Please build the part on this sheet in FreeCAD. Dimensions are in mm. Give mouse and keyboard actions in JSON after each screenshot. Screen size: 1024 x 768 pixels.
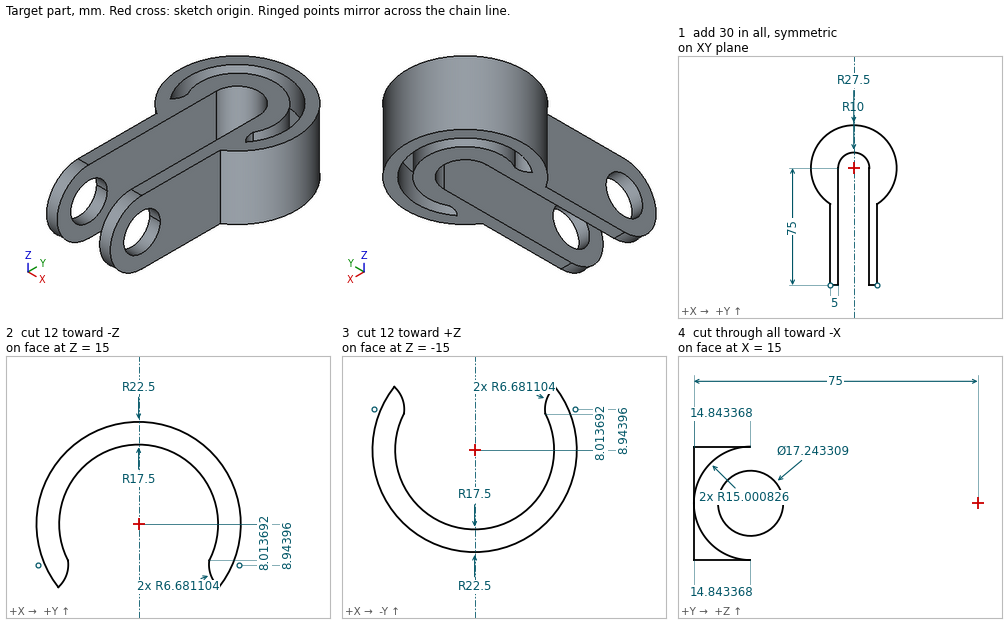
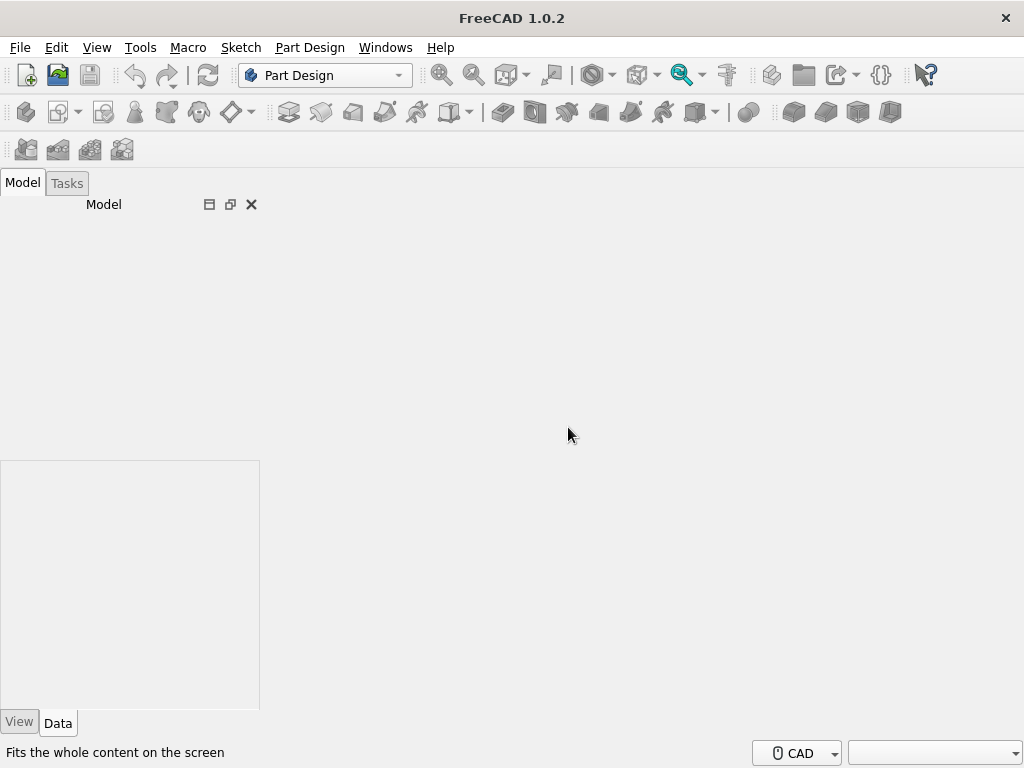
{"action": "left_click", "coordinate": [26, 76]}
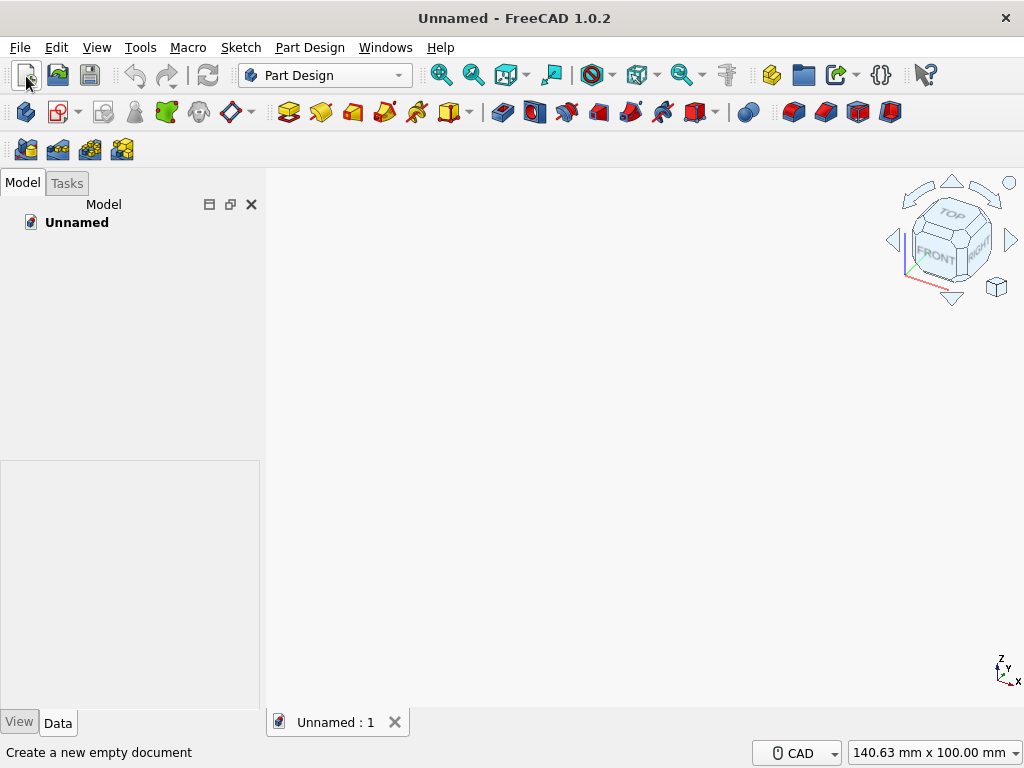
{"action": "left_click", "coordinate": [58, 112]}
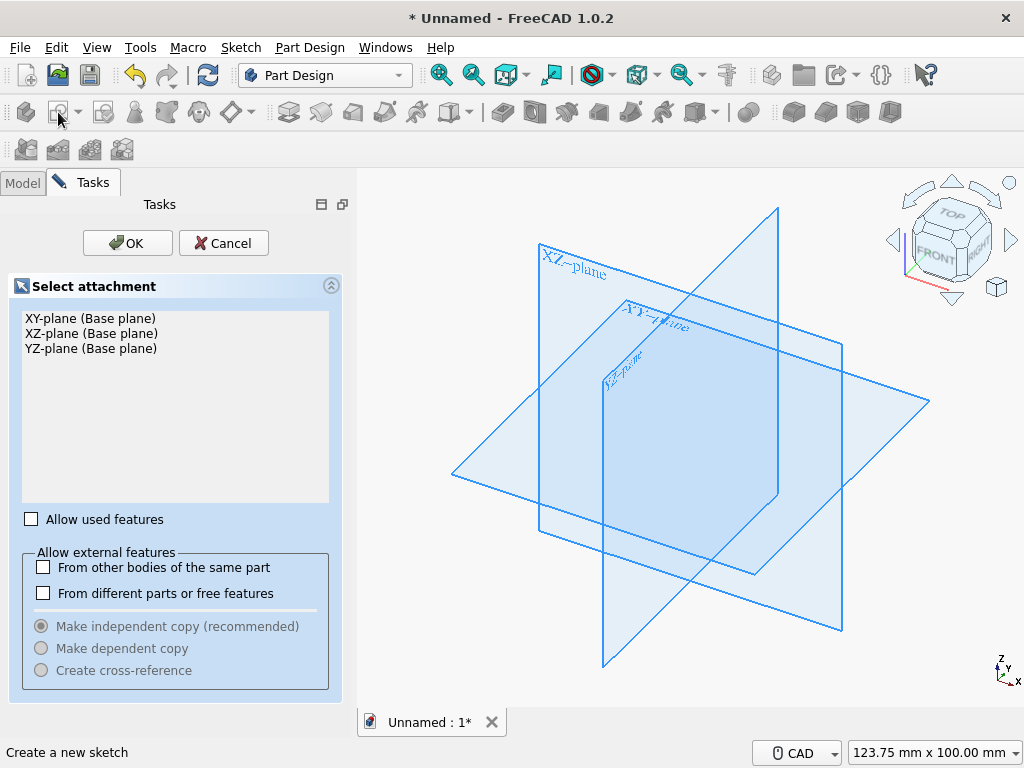
{"action": "left_click", "coordinate": [82, 318]}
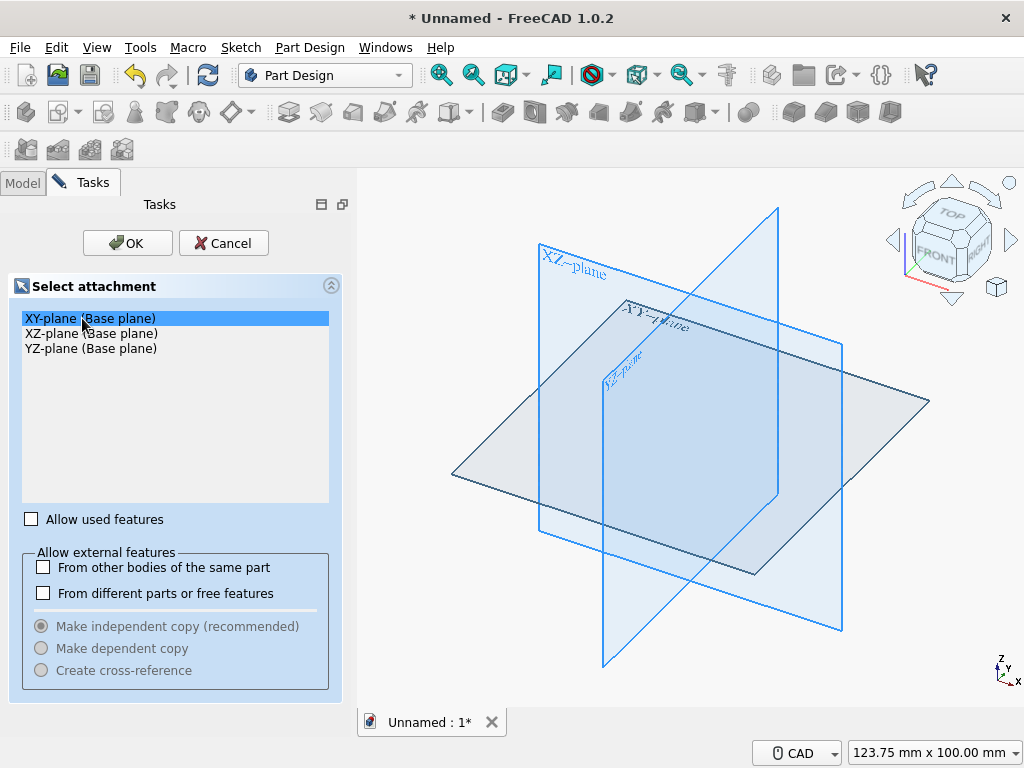
{"action": "left_click", "coordinate": [128, 243]}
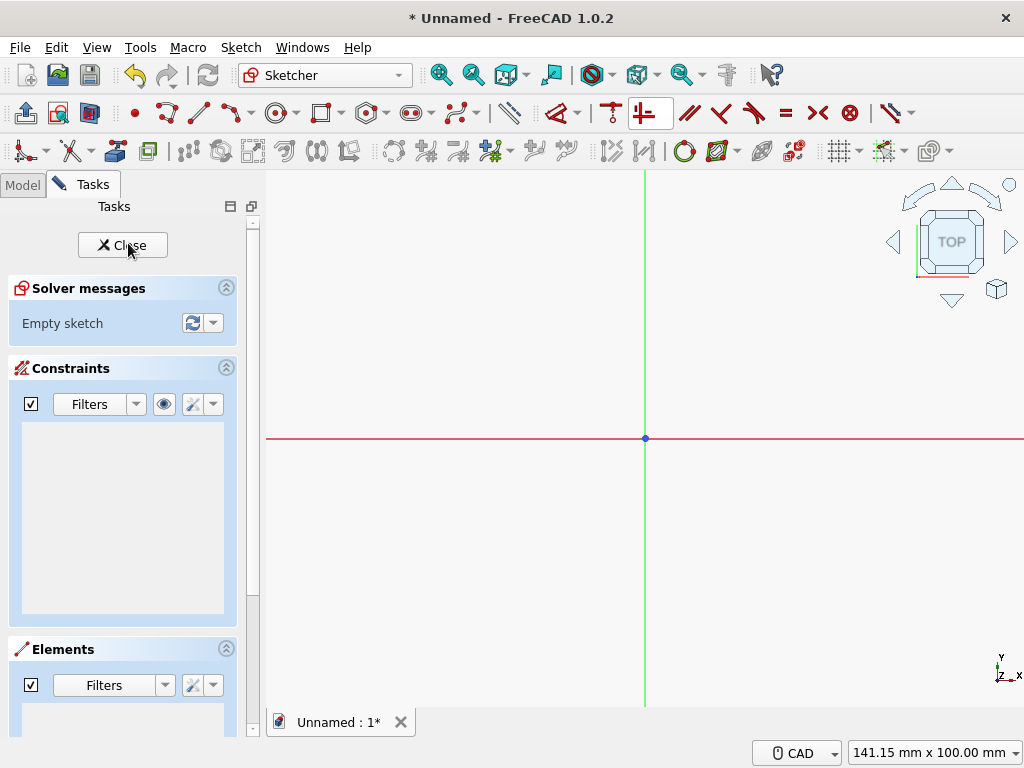
{"action": "scroll", "coordinate": [437, 198], "scroll_direction": "down", "scroll_amount": 2}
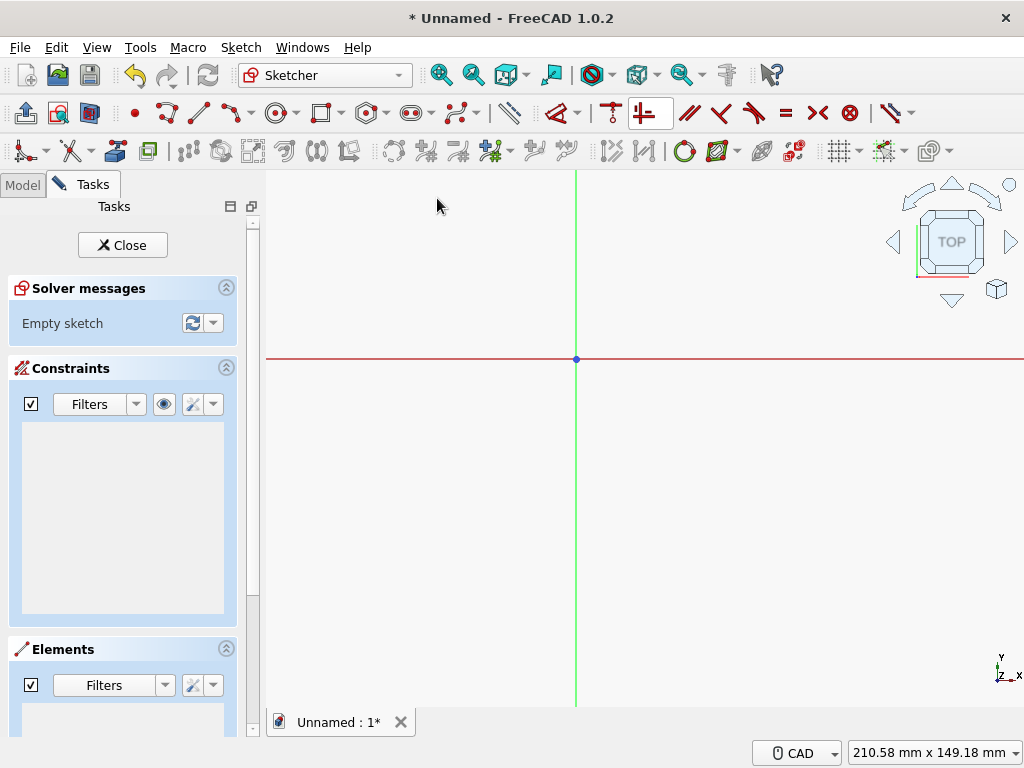
{"action": "key", "text": "g m"}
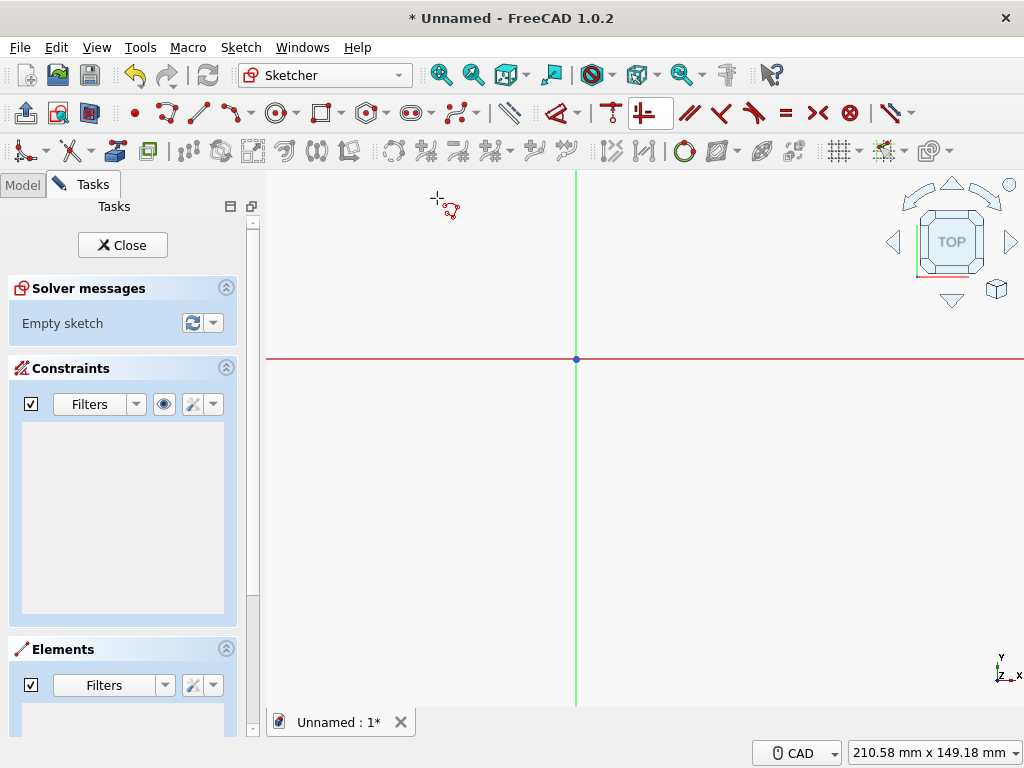
{"action": "left_click", "coordinate": [523, 442]}
{"action": "left_click", "coordinate": [523, 629]}
{"action": "left_click", "coordinate": [541, 629]}
{"action": "left_click", "coordinate": [541, 359]}
{"action": "right_click", "coordinate": [541, 359]}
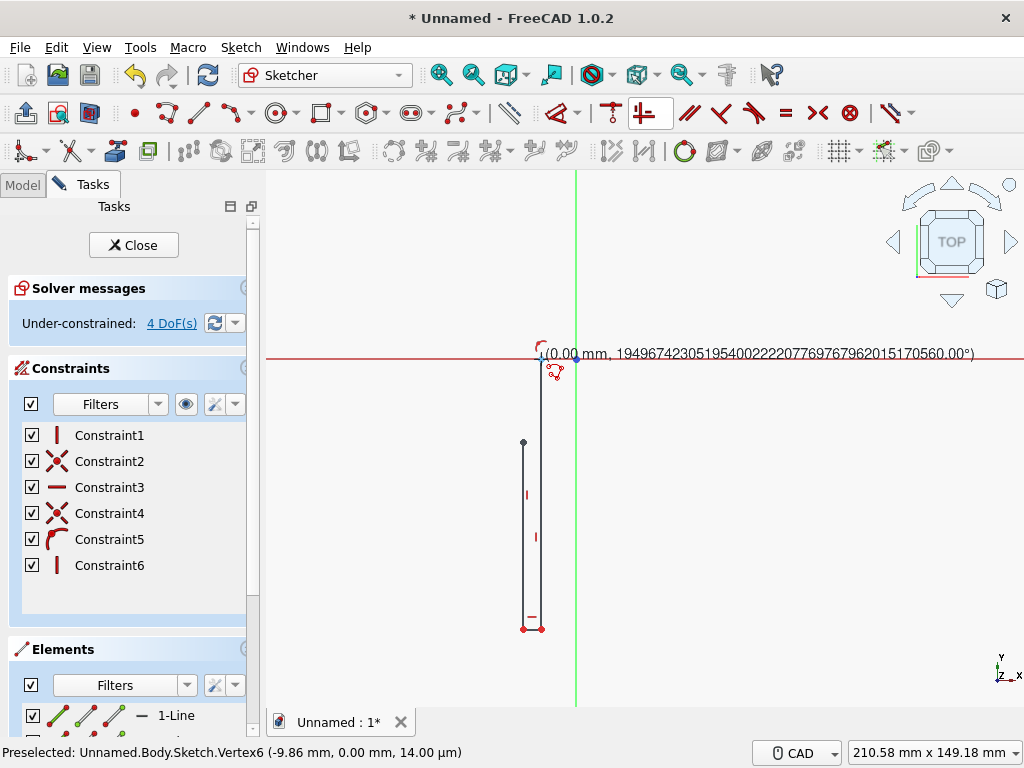
{"action": "left_click", "coordinate": [612, 359]}
{"action": "left_click", "coordinate": [612, 629]}
{"action": "left_click", "coordinate": [630, 629]}
{"action": "left_click", "coordinate": [630, 442]}
{"action": "right_click", "coordinate": [630, 442]}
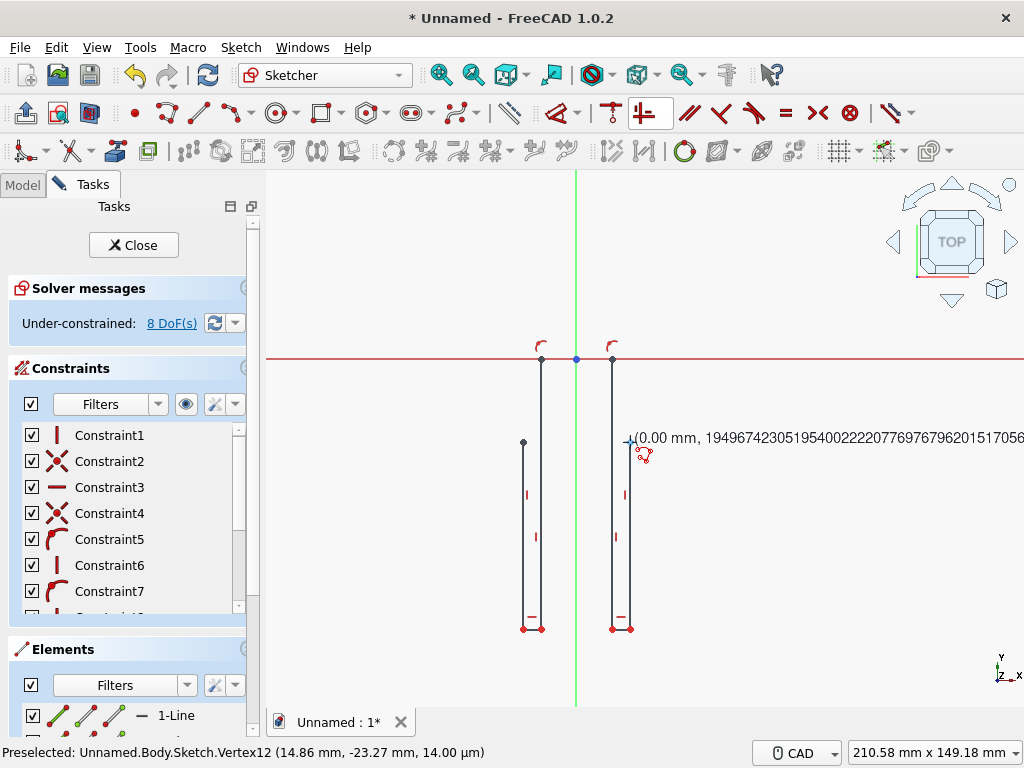
{"action": "key", "text": "g 3 a"}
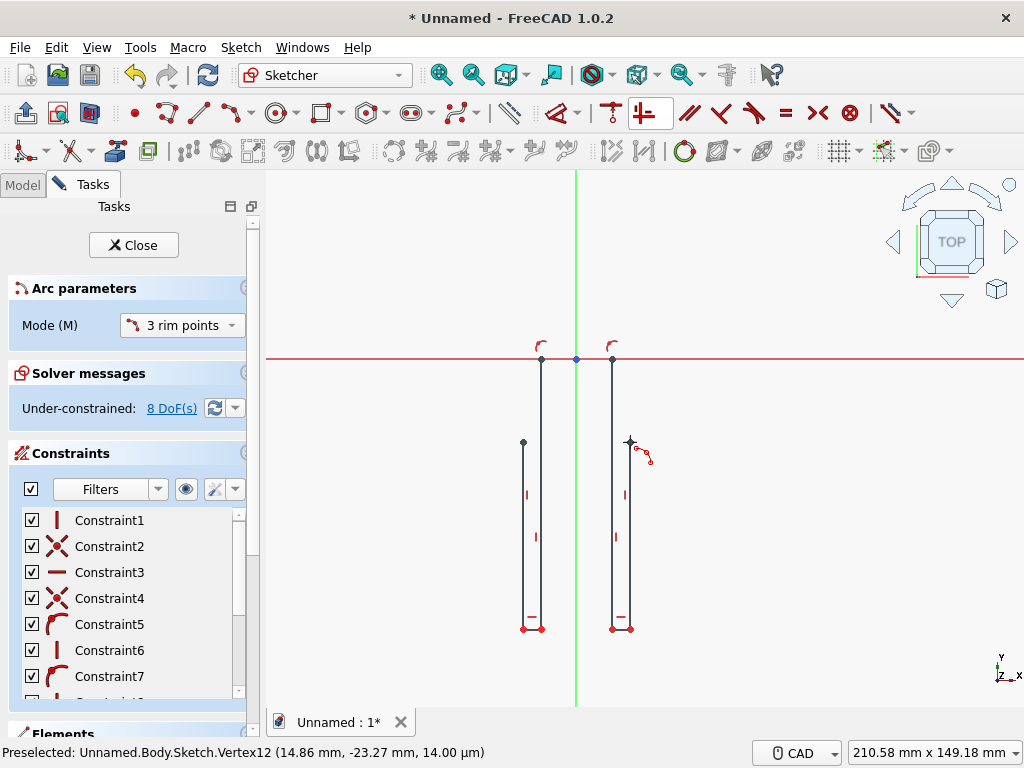
{"action": "left_click", "coordinate": [541, 359]}
{"action": "left_click", "coordinate": [612, 359]}
{"action": "left_click", "coordinate": [598, 330]}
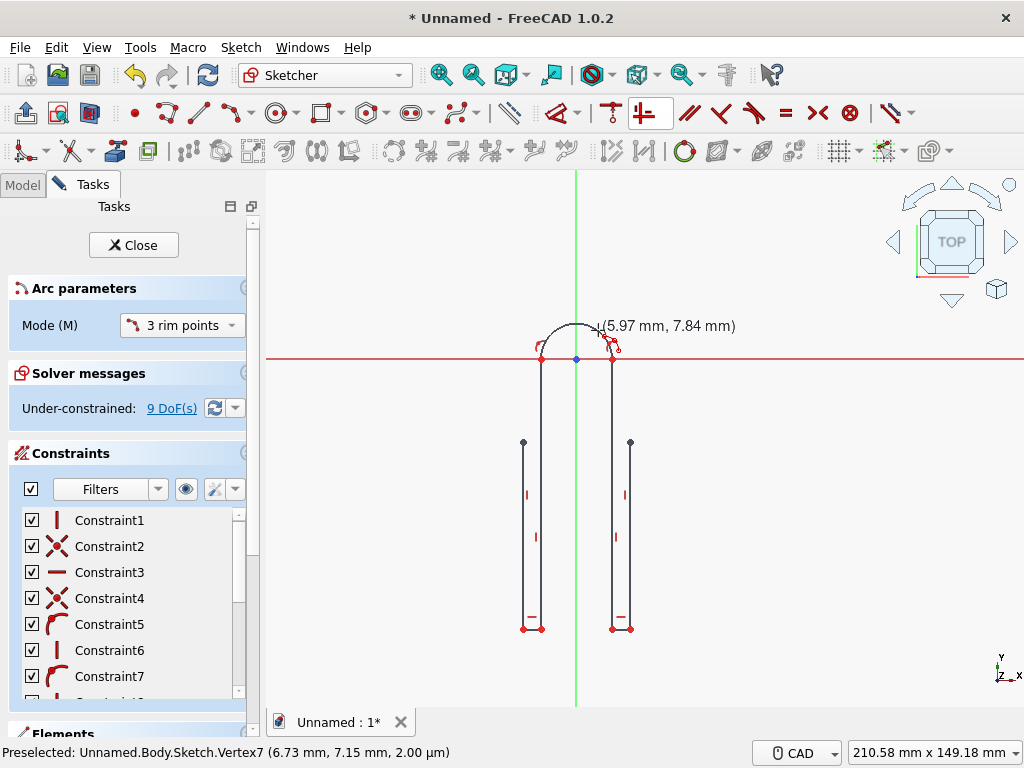
{"action": "left_click", "coordinate": [630, 443]}
{"action": "left_click", "coordinate": [523, 443]}
{"action": "left_click", "coordinate": [625, 273]}
{"action": "key", "text": "Escape"}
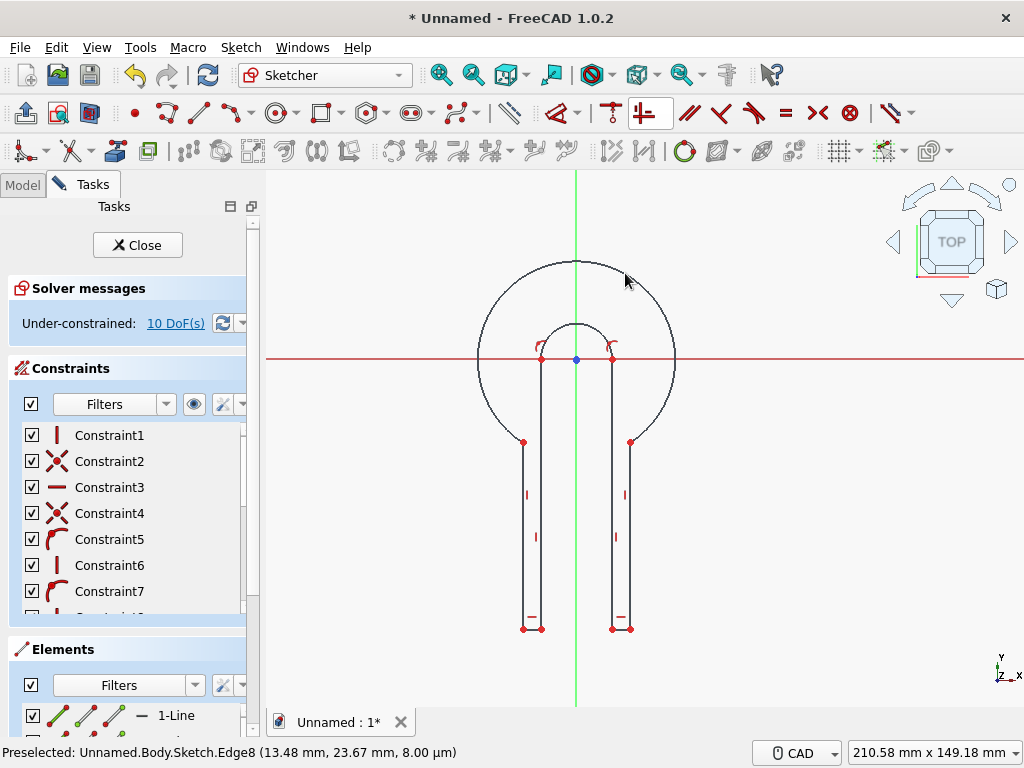
{"action": "left_click", "coordinate": [541, 549]}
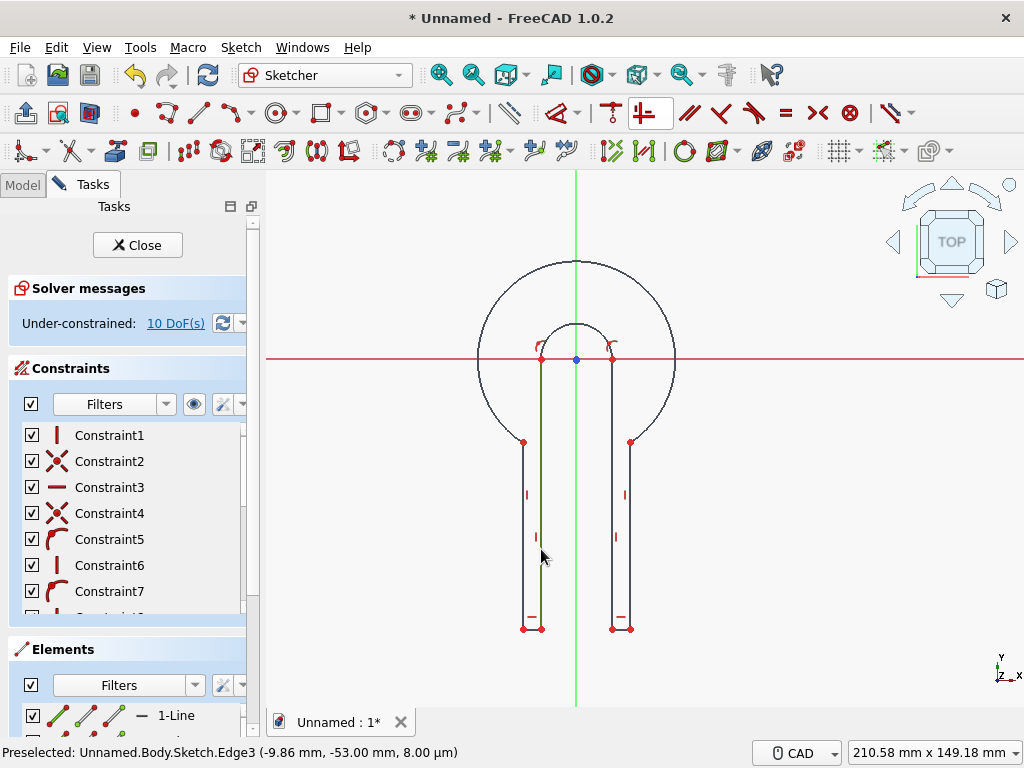
{"action": "left_click", "coordinate": [597, 331]}